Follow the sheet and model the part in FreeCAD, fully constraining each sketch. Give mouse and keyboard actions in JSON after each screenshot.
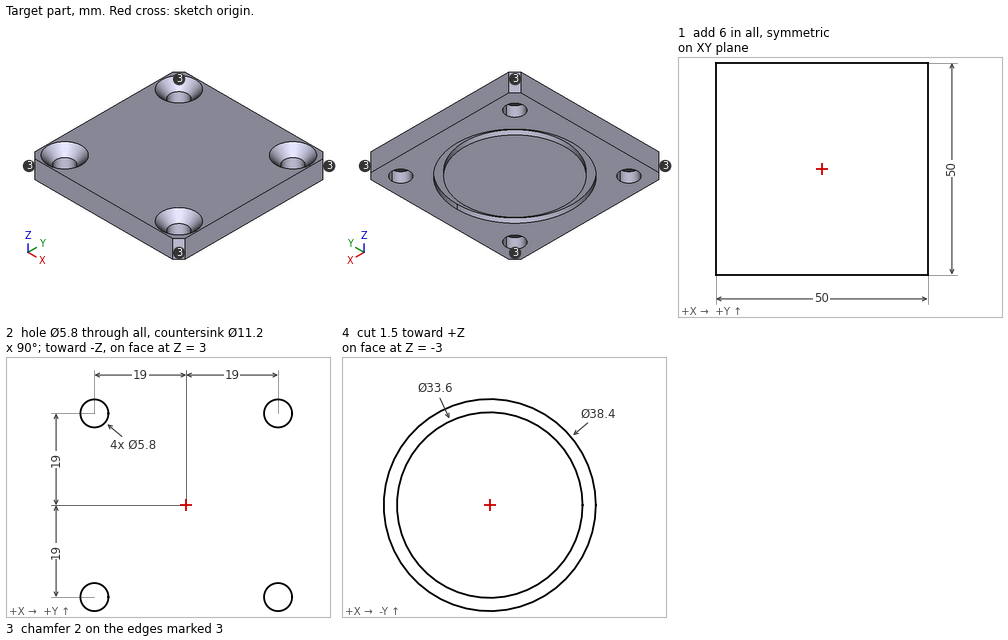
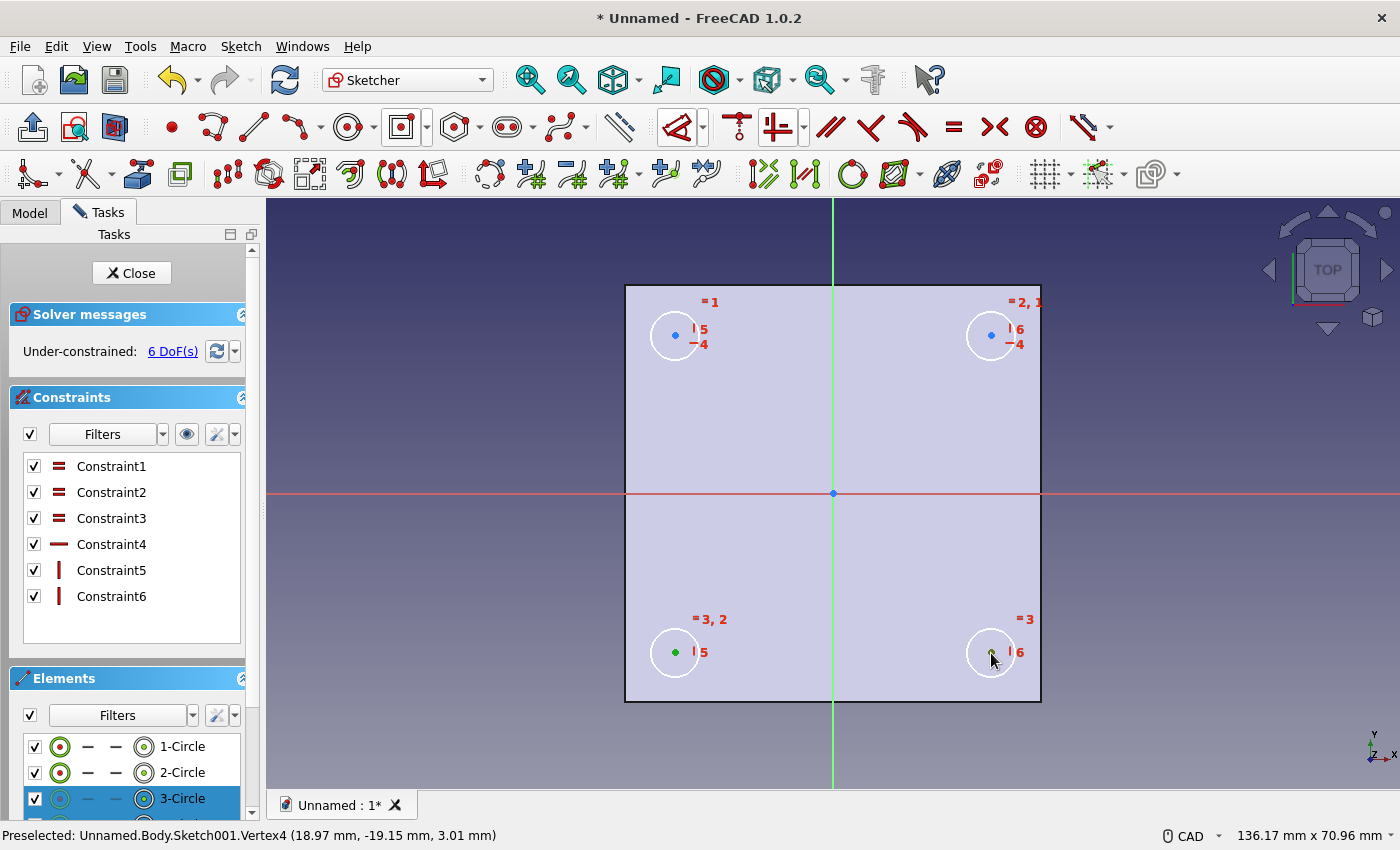
{"action": "left_click", "coordinate": [804, 128]}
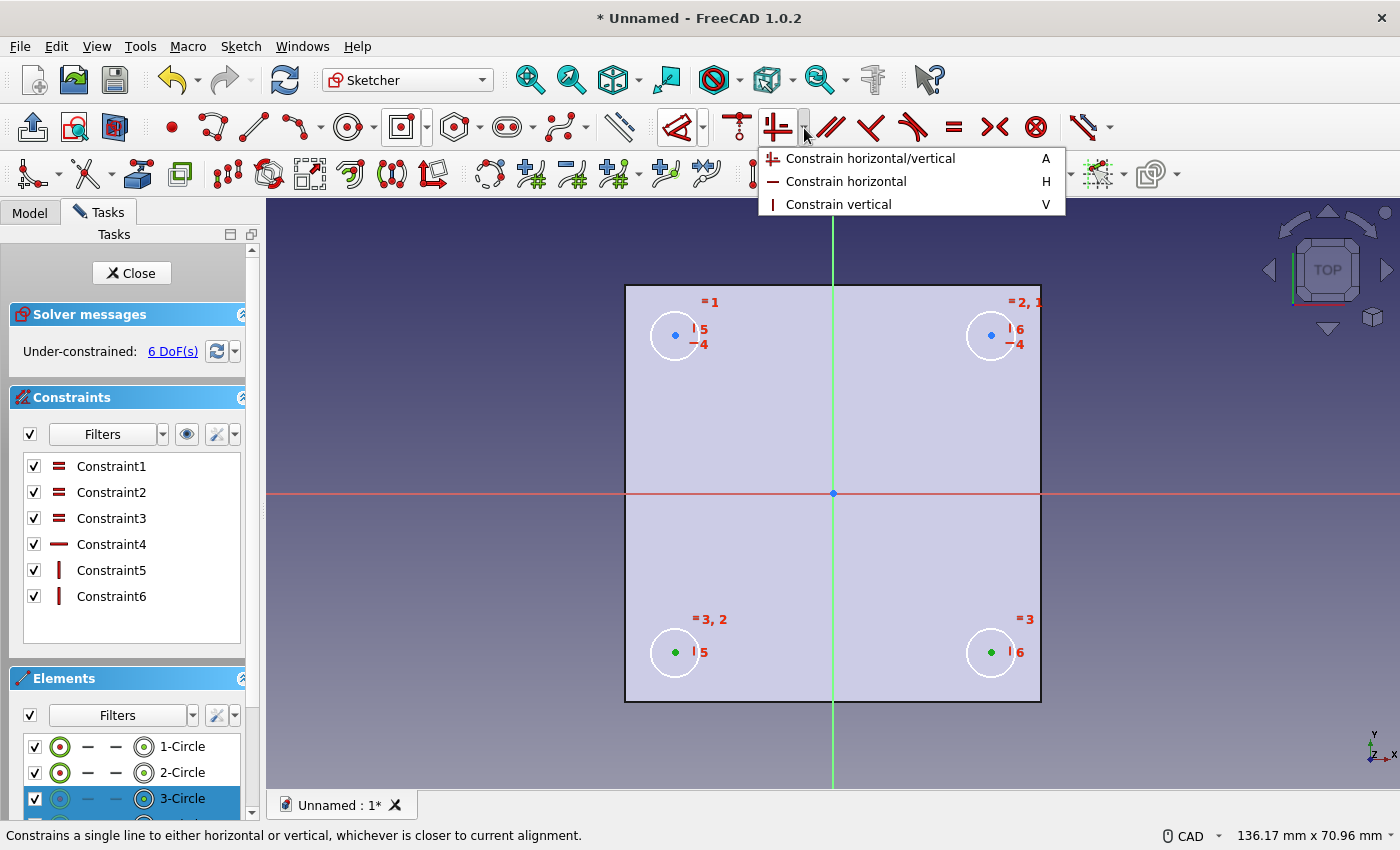
{"action": "left_click", "coordinate": [912, 182]}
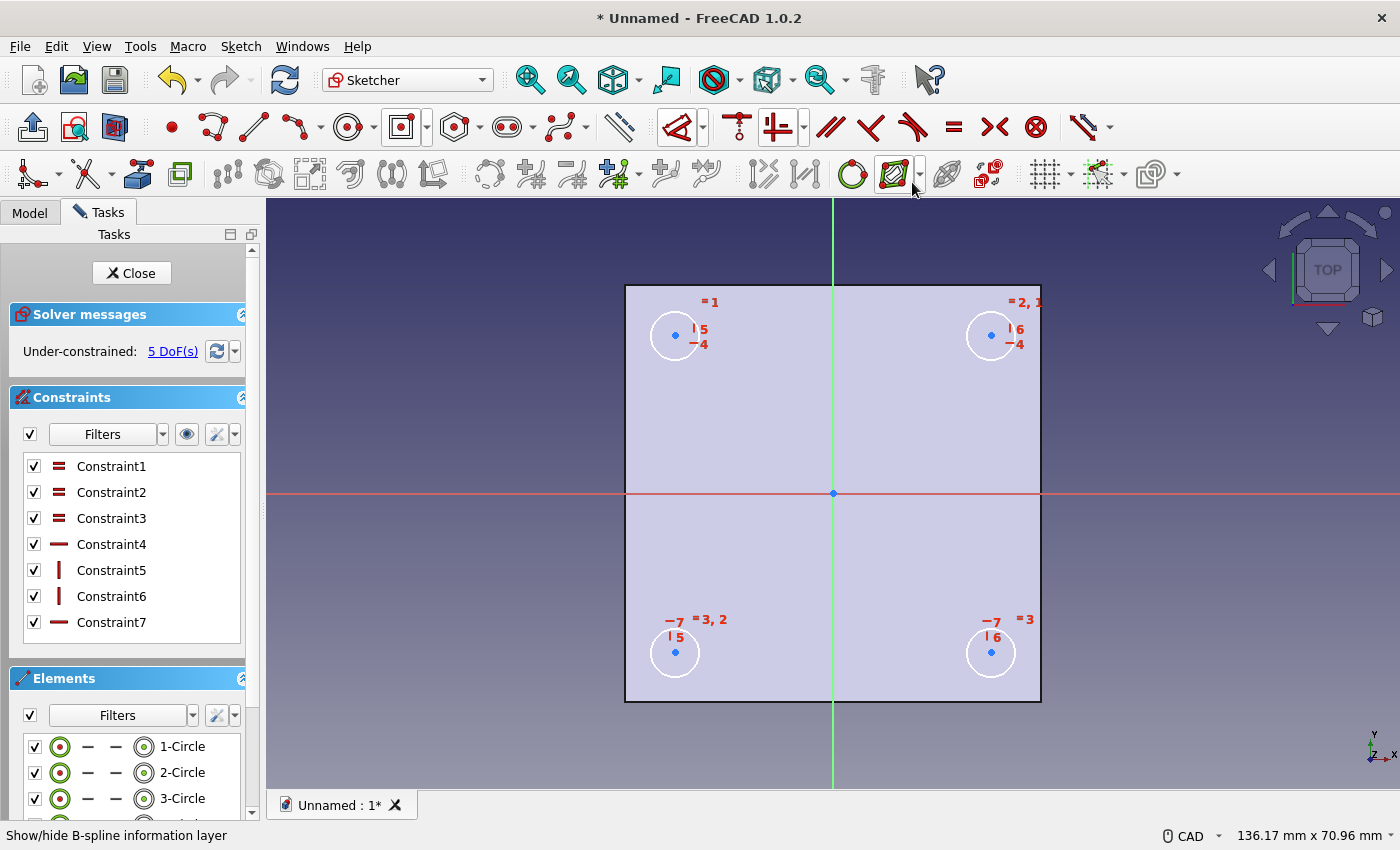
{"action": "left_click", "coordinate": [692, 319]}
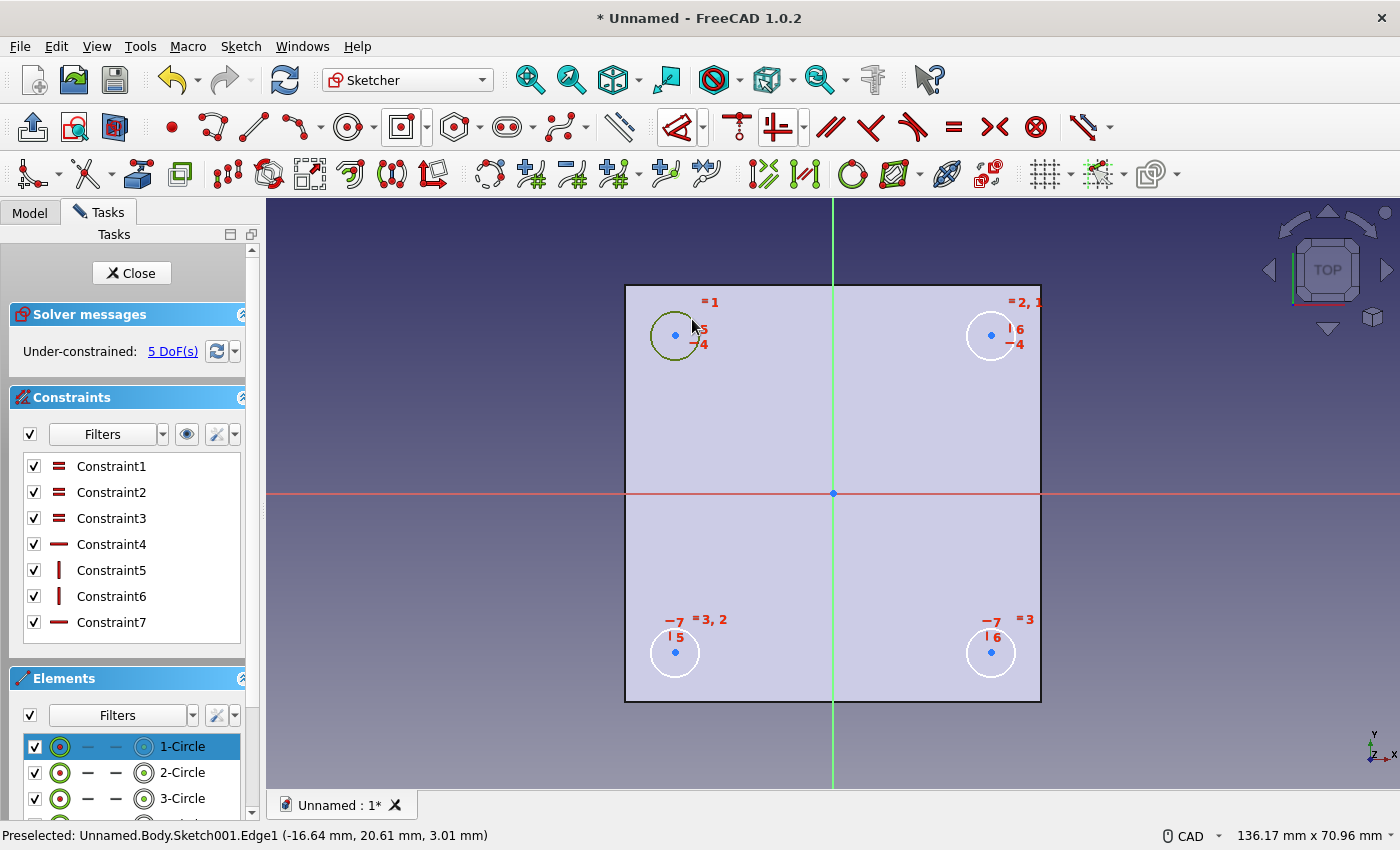
{"action": "left_click", "coordinate": [702, 128]}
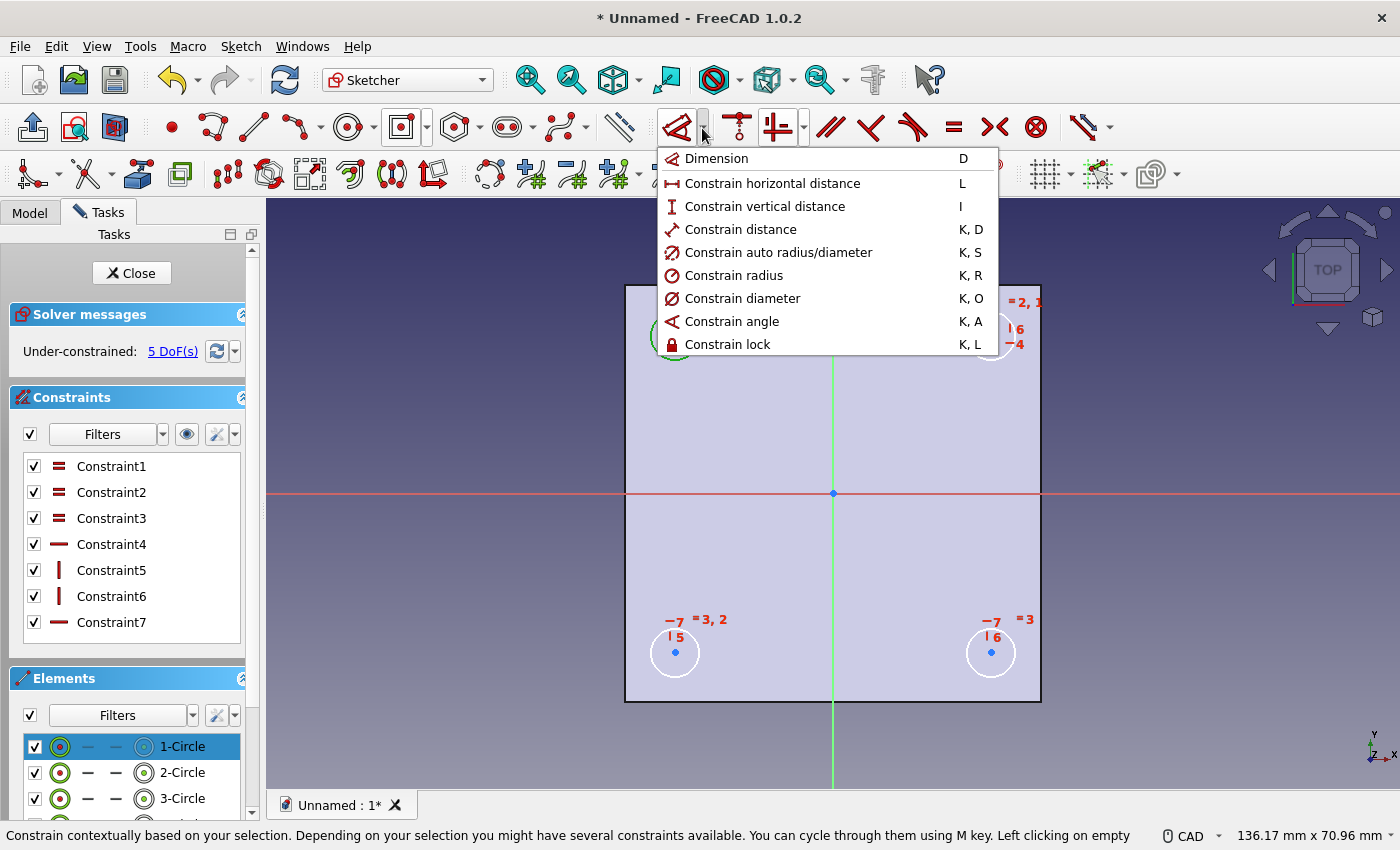
{"action": "left_click", "coordinate": [828, 298]}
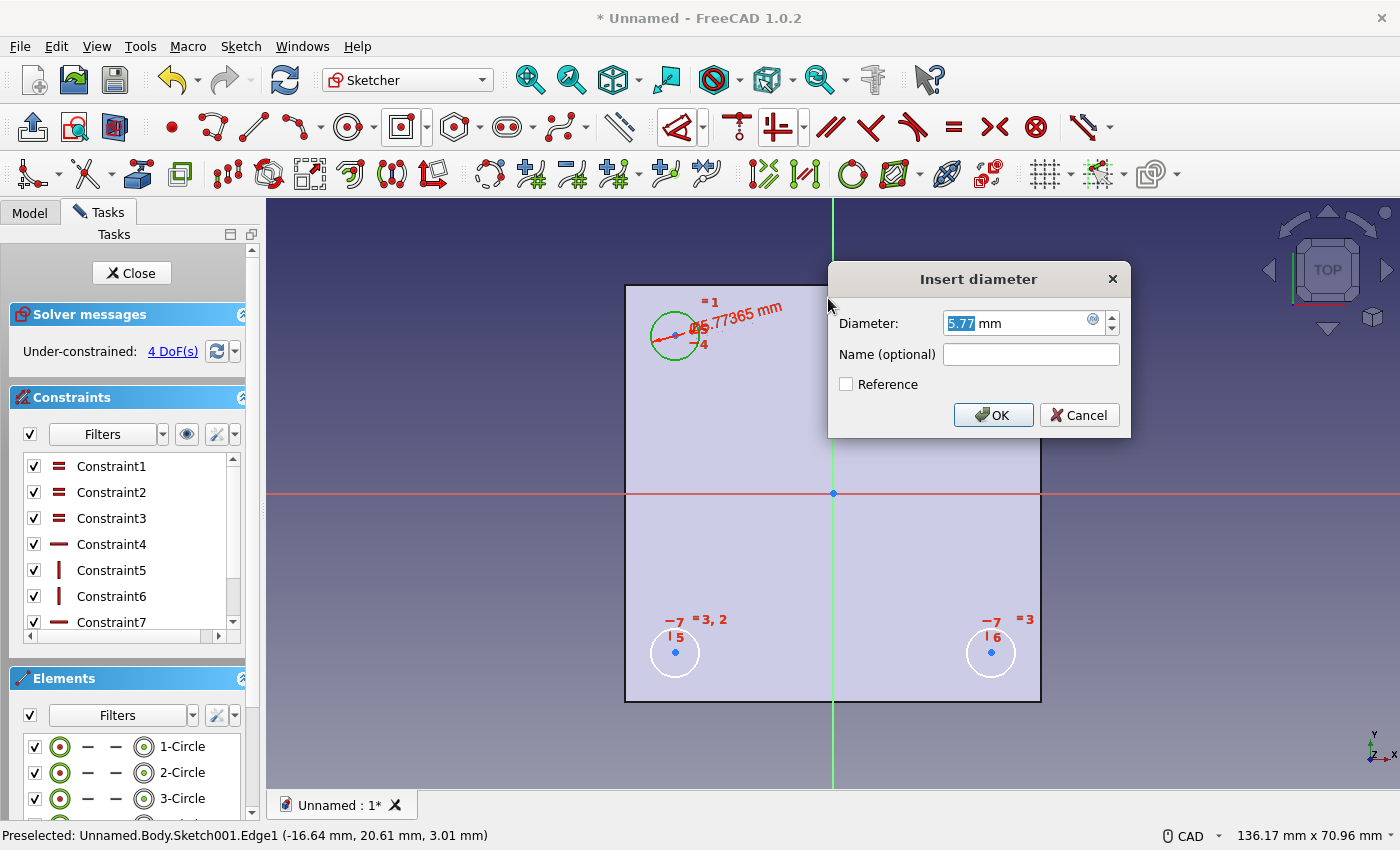
{"action": "type", "text": "5.8"}
{"action": "key", "text": "Return"}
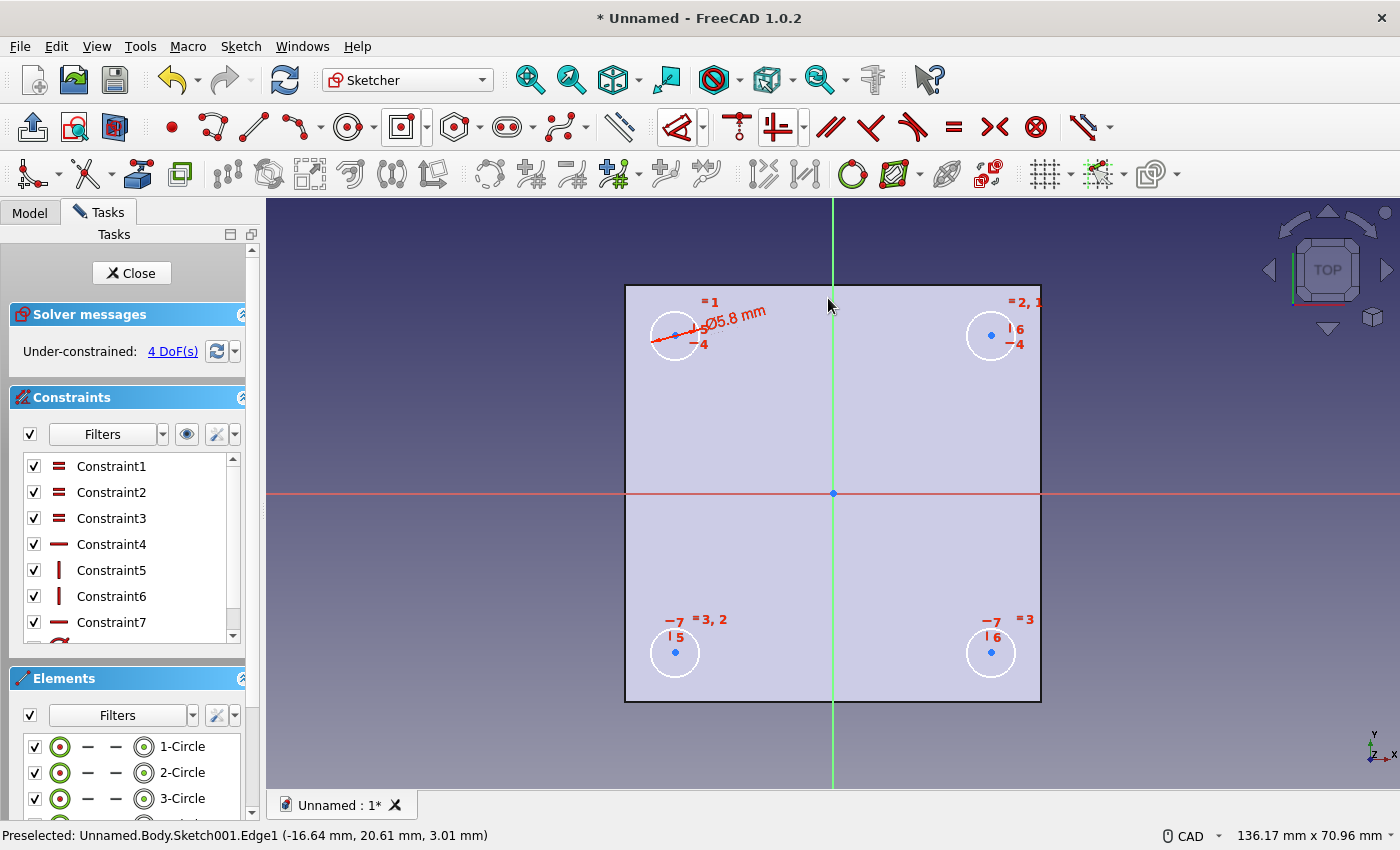
{"action": "left_click", "coordinate": [675, 336]}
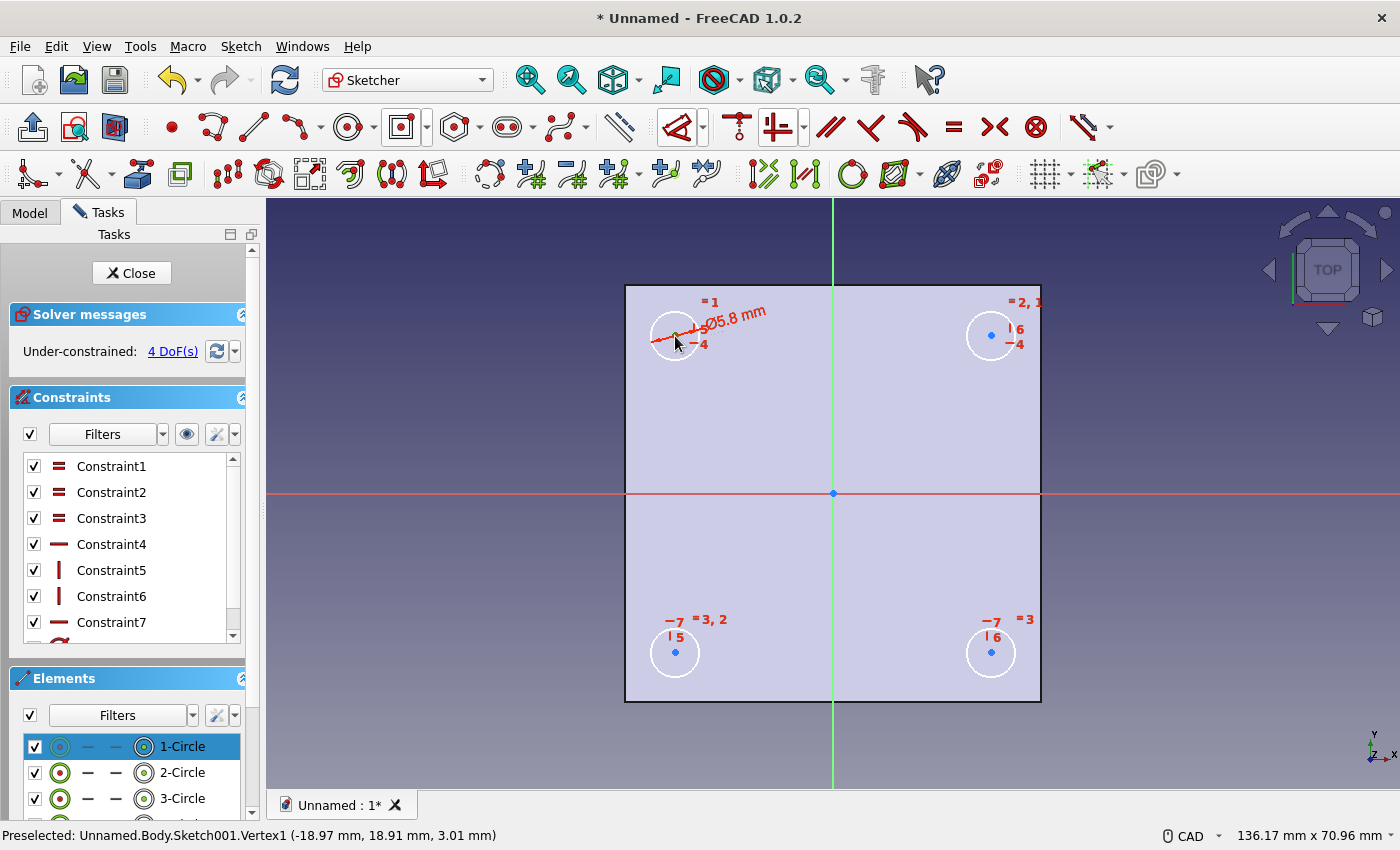
{"action": "left_click", "coordinate": [702, 128]}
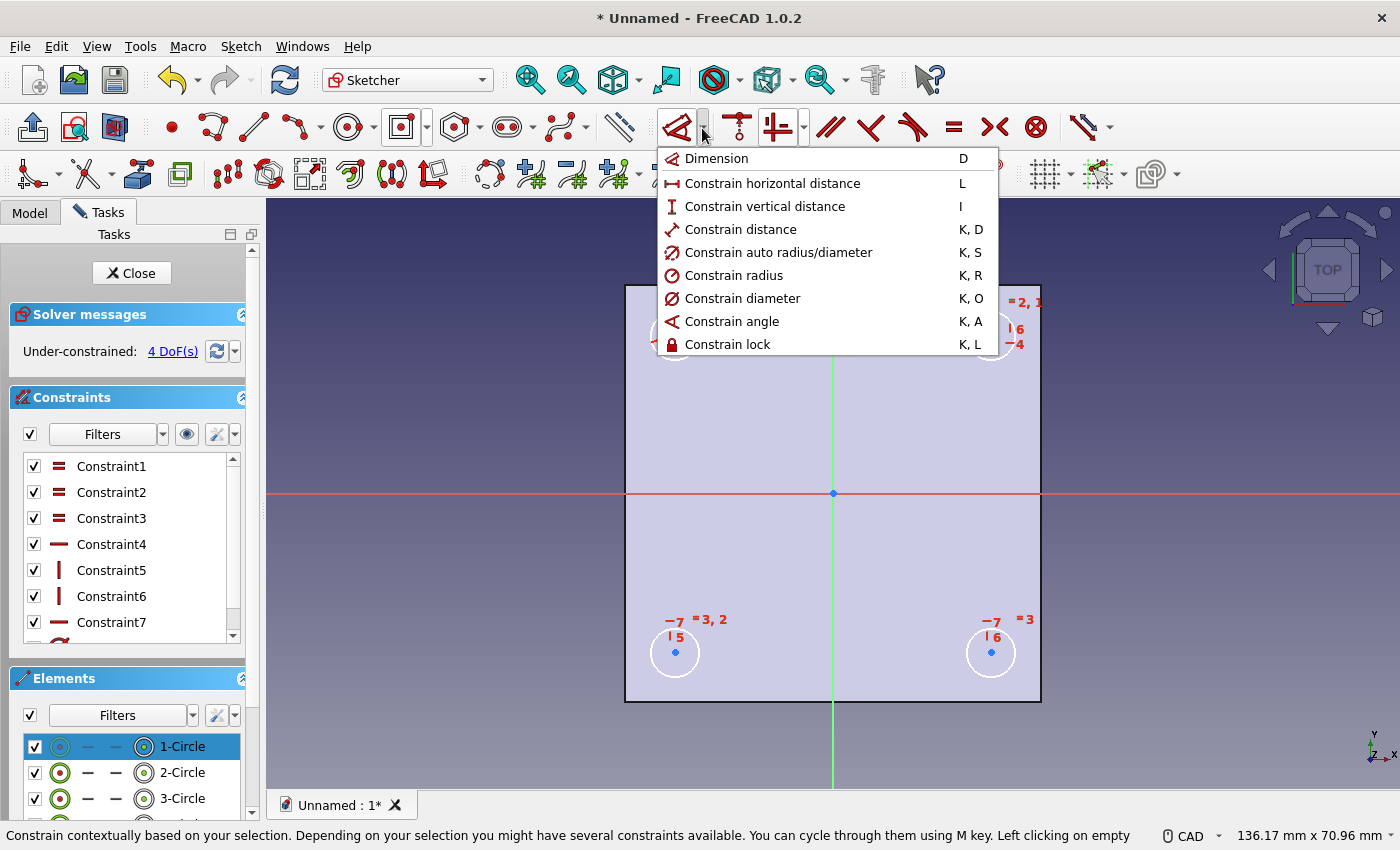
{"action": "left_click", "coordinate": [828, 184]}